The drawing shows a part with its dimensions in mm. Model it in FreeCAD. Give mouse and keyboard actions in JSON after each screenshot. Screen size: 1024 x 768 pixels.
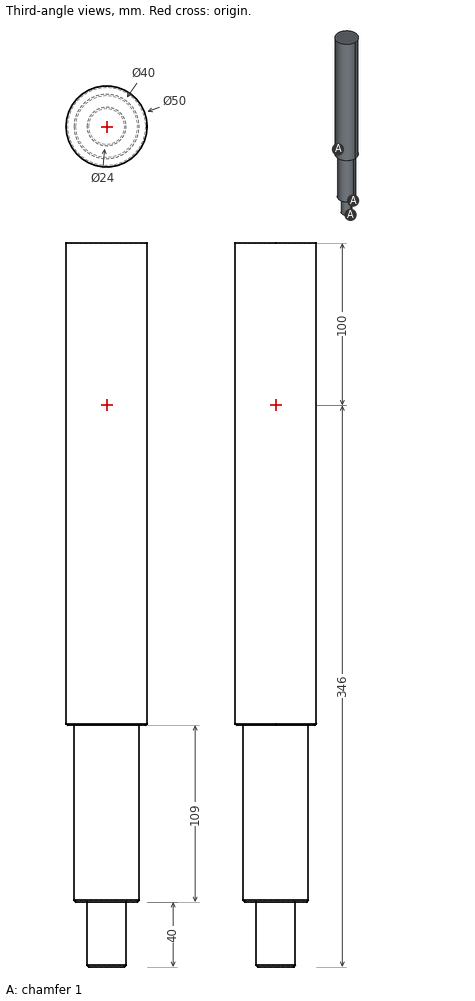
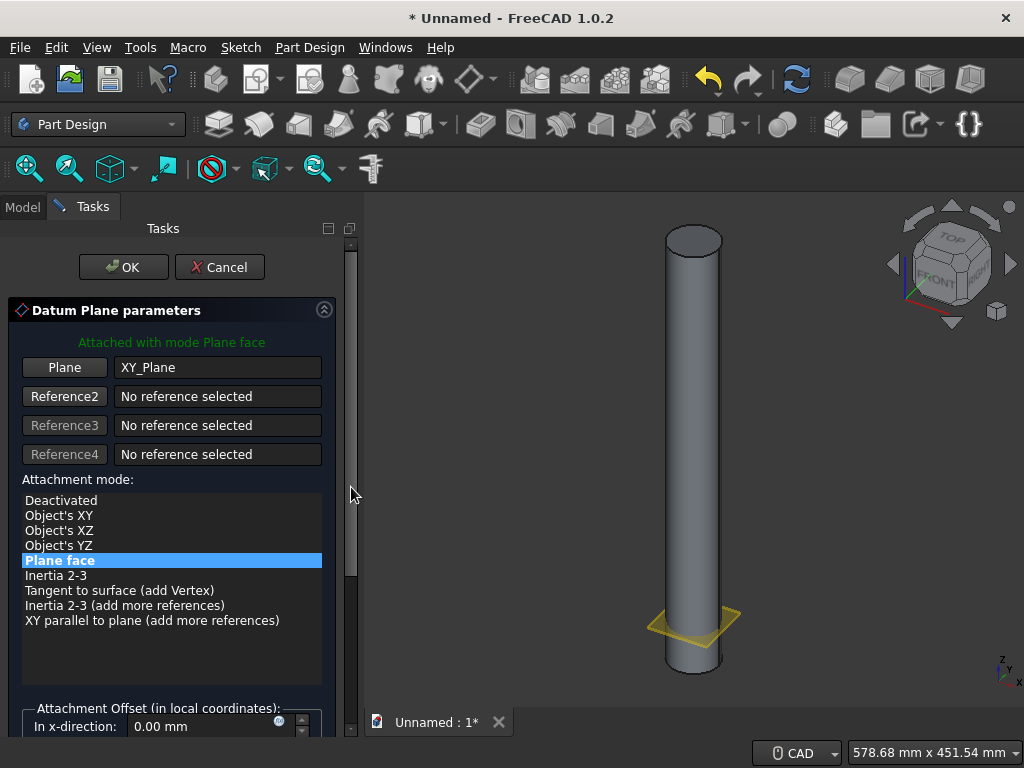
{"action": "left_click", "coordinate": [124, 267]}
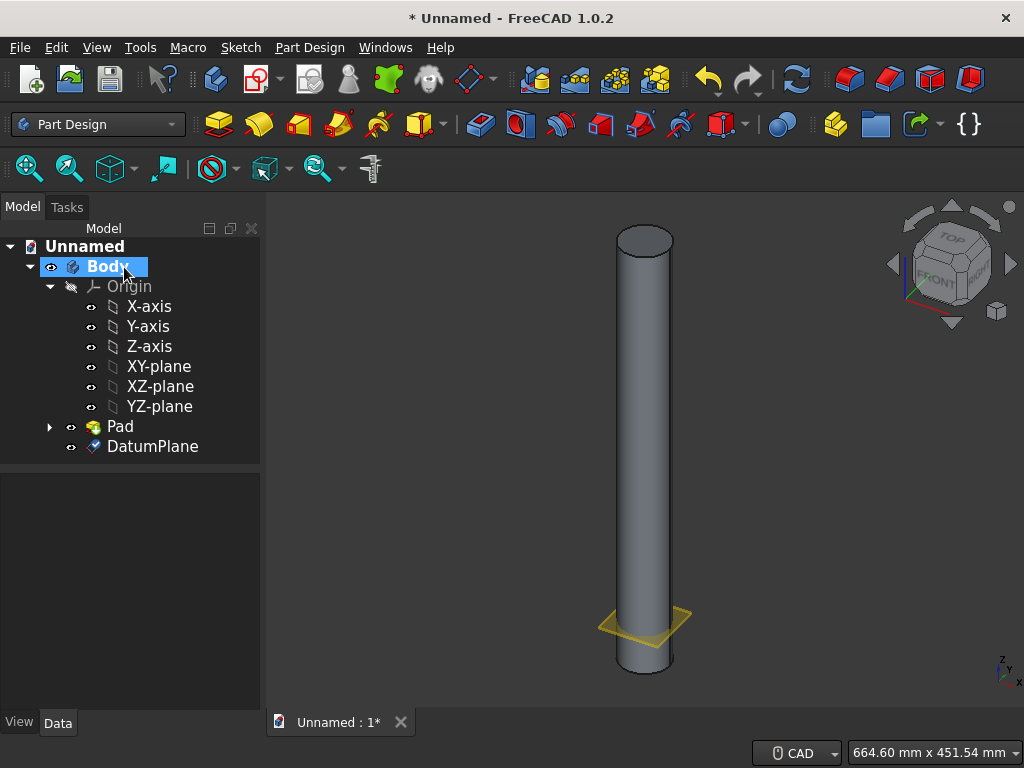
{"action": "left_click", "coordinate": [116, 447]}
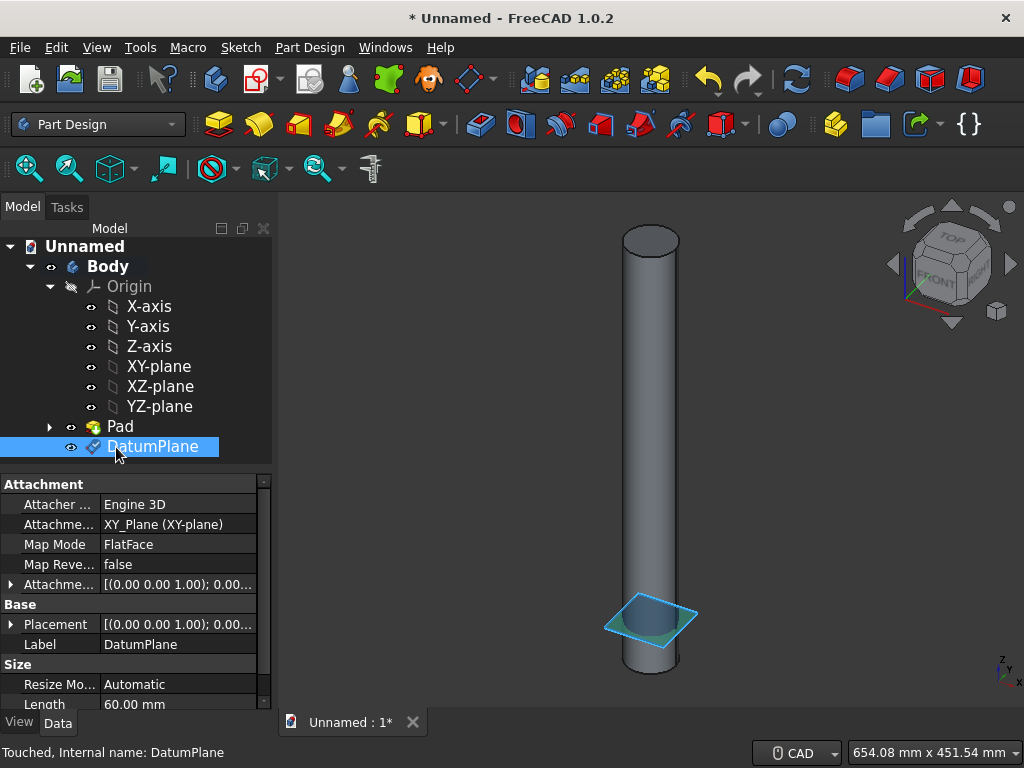
{"action": "left_click", "coordinate": [256, 80]}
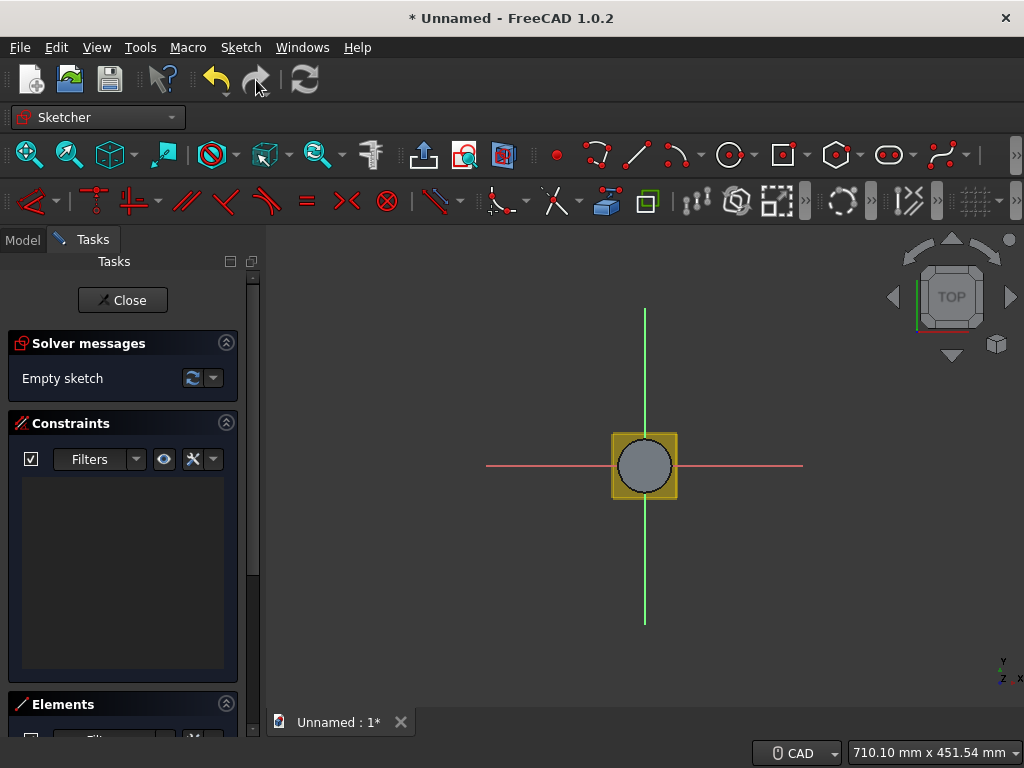
{"action": "left_click", "coordinate": [504, 156]}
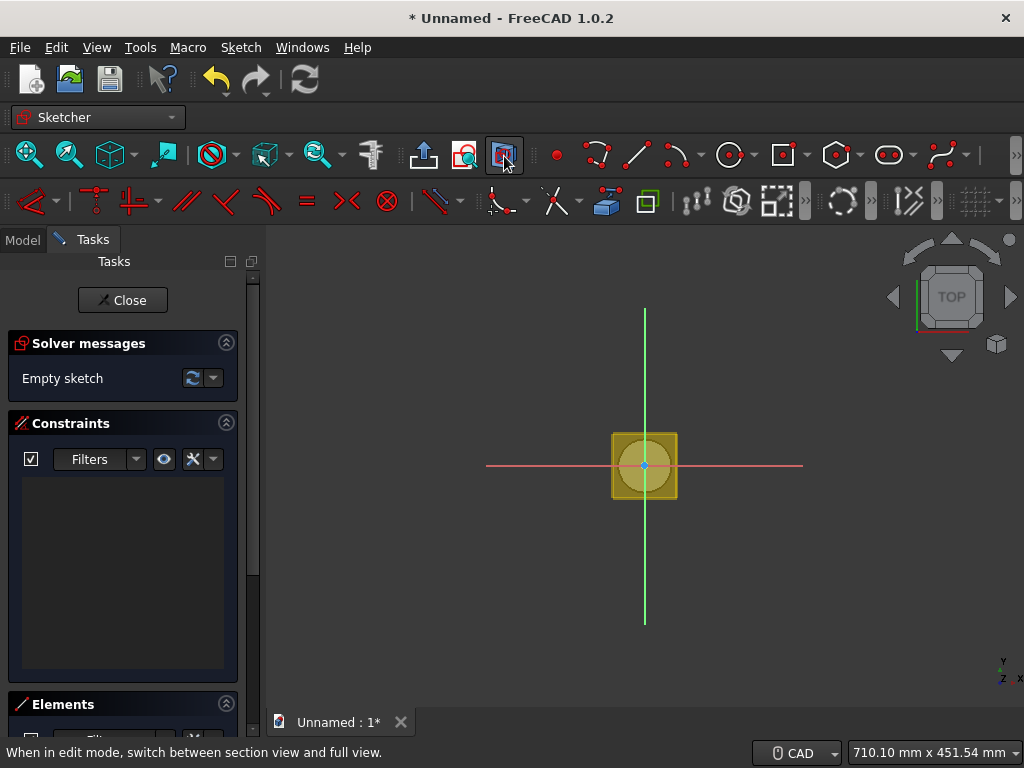
{"action": "scroll", "coordinate": [658, 466], "scroll_direction": "up", "scroll_amount": 9}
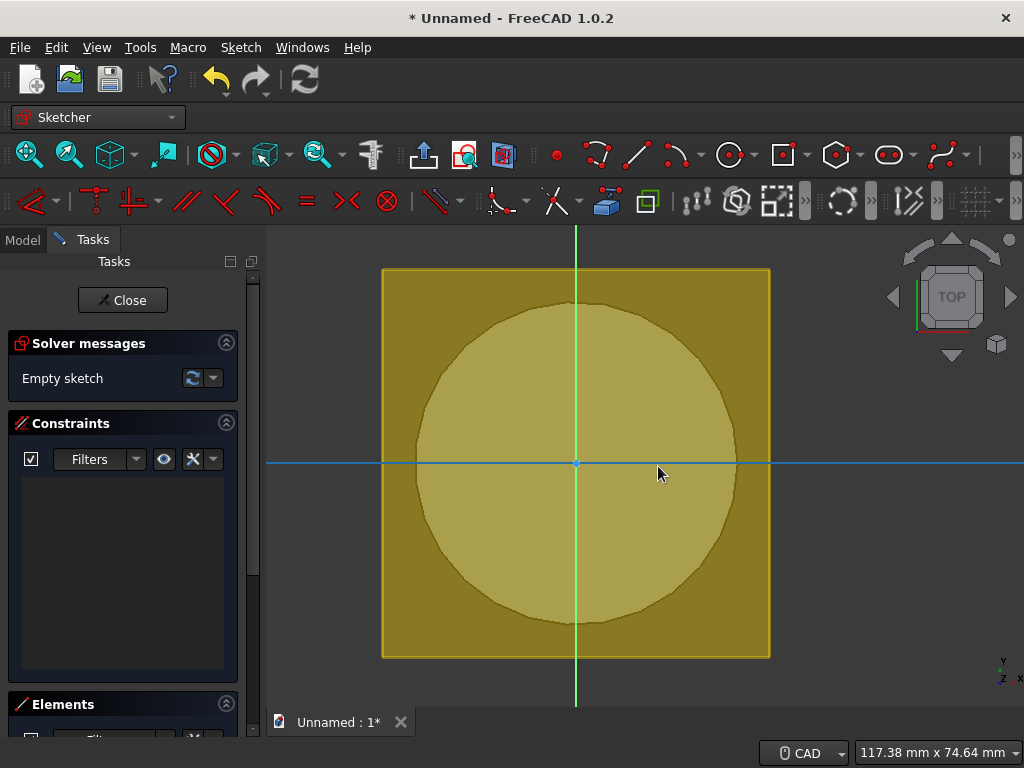
{"action": "left_click", "coordinate": [730, 156]}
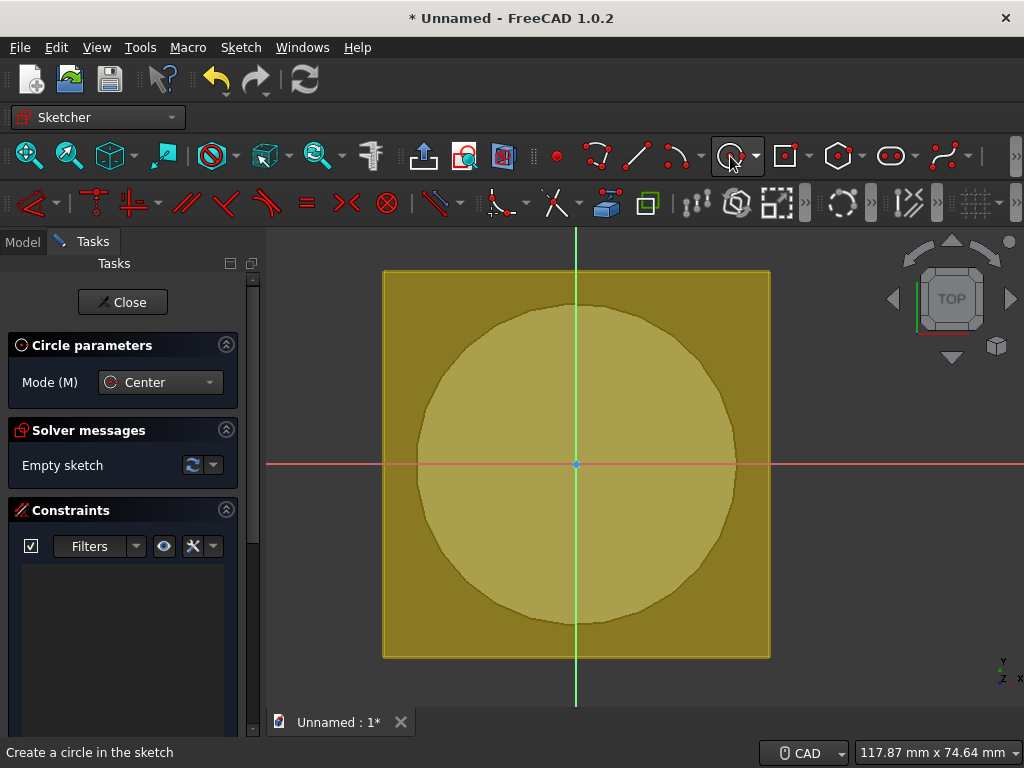
{"action": "left_click", "coordinate": [576, 464]}
{"action": "left_click", "coordinate": [690, 351]}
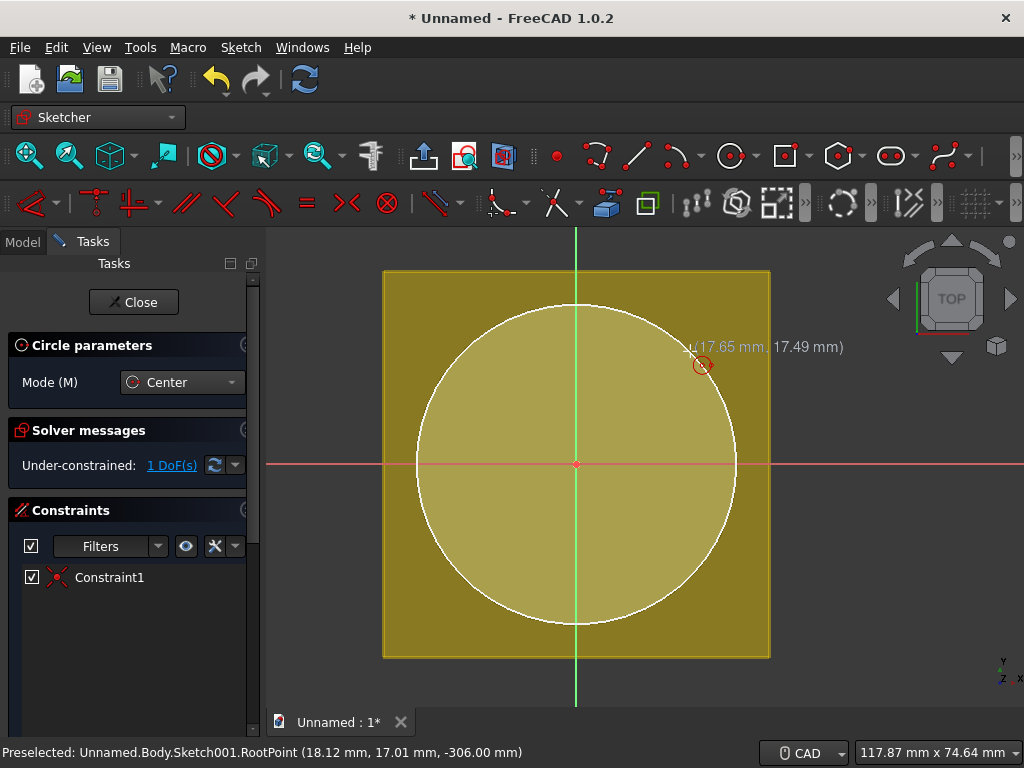
{"action": "left_click", "coordinate": [576, 464]}
{"action": "left_click", "coordinate": [667, 374]}
{"action": "key", "text": "Escape"}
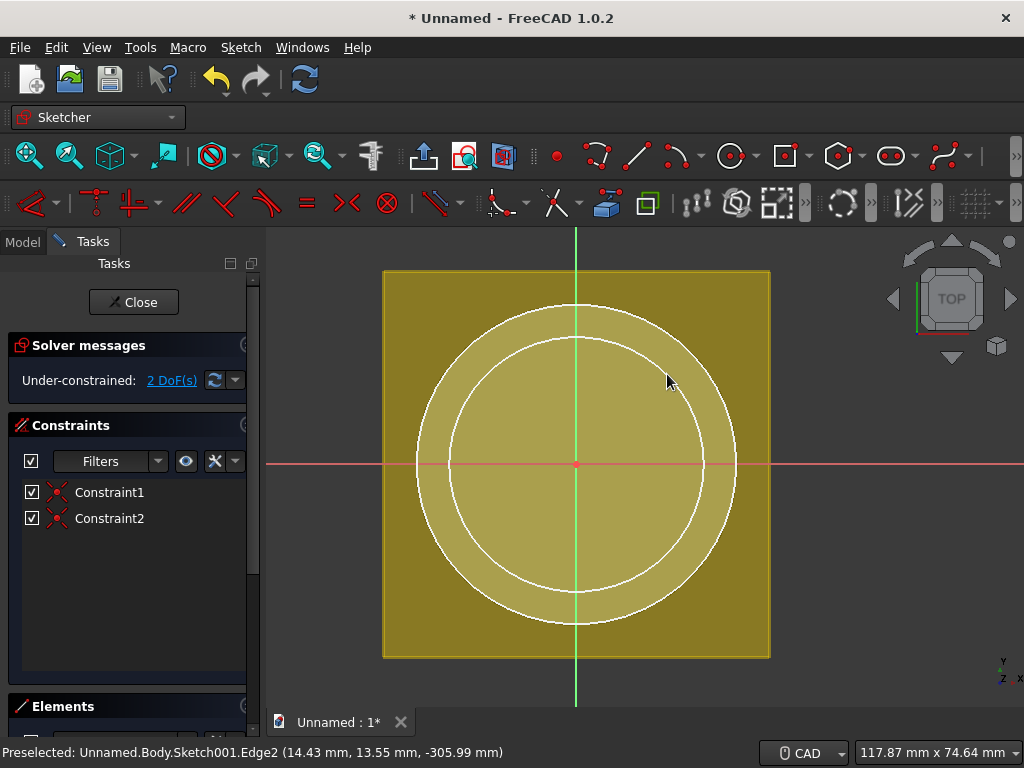
{"action": "key", "text": "d"}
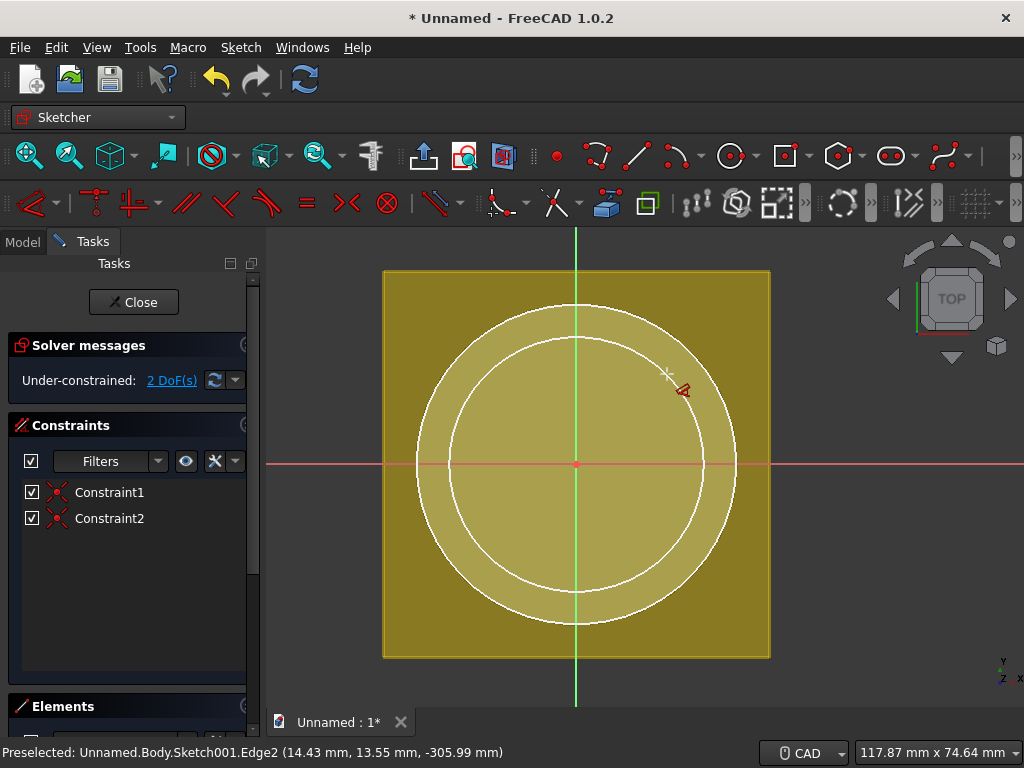
{"action": "left_click", "coordinate": [689, 351]}
{"action": "left_click", "coordinate": [712, 328]}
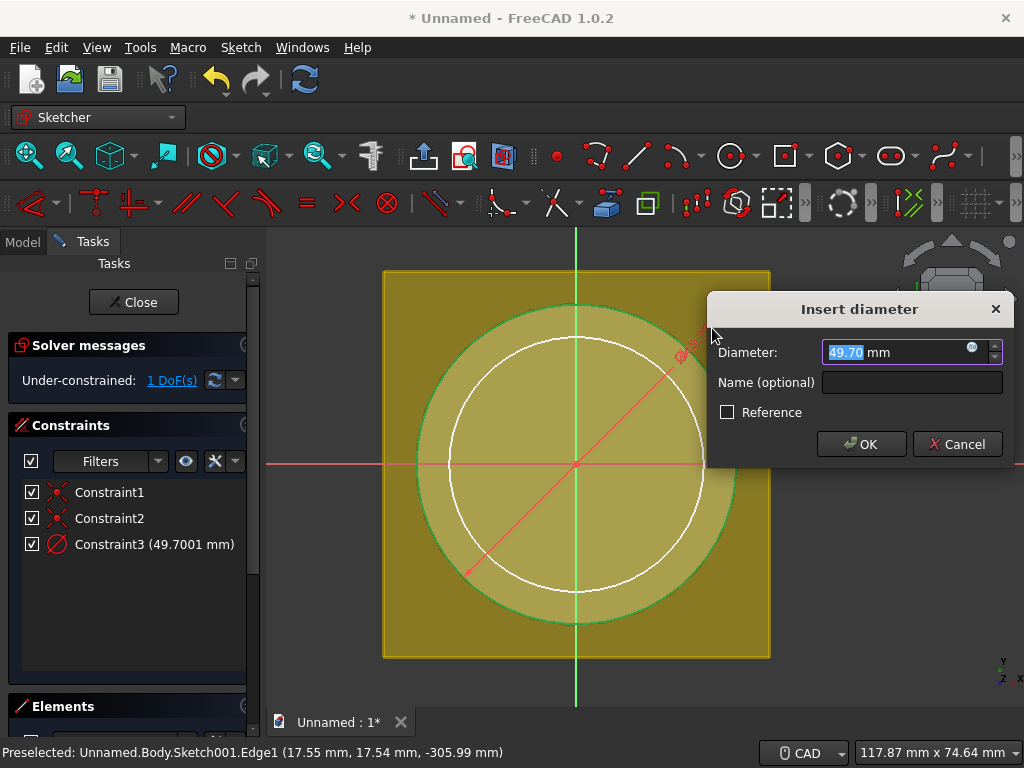
{"action": "type", "text": "50"}
{"action": "key", "text": "Return"}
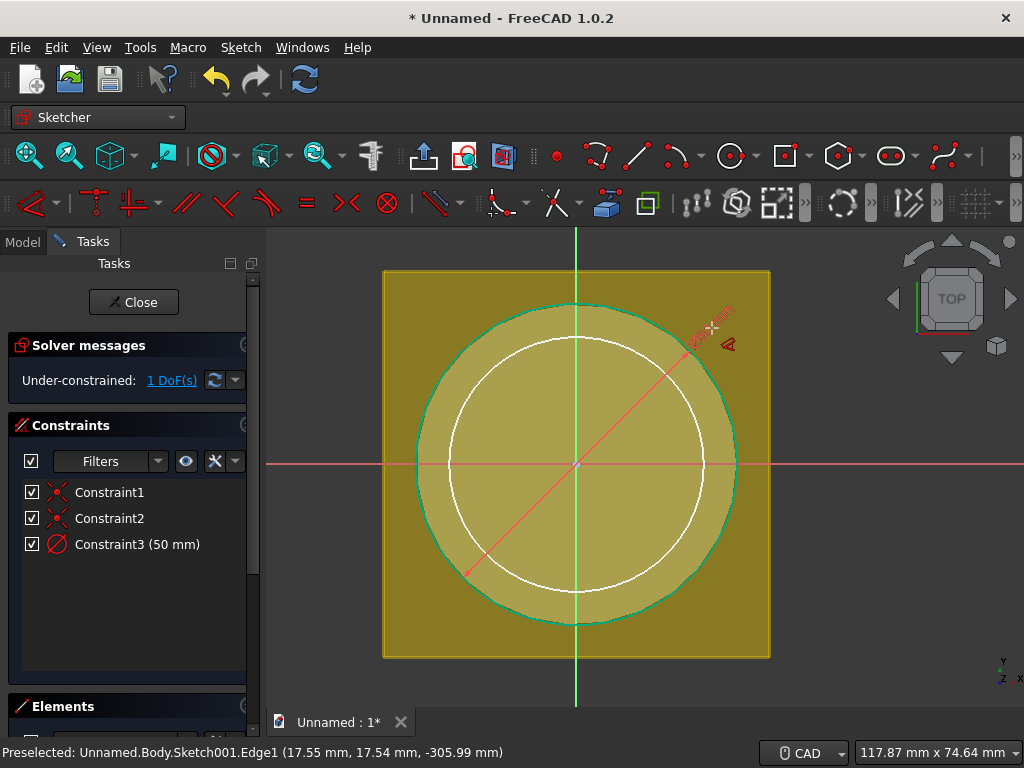
{"action": "left_click", "coordinate": [666, 374]}
{"action": "left_click", "coordinate": [751, 412]}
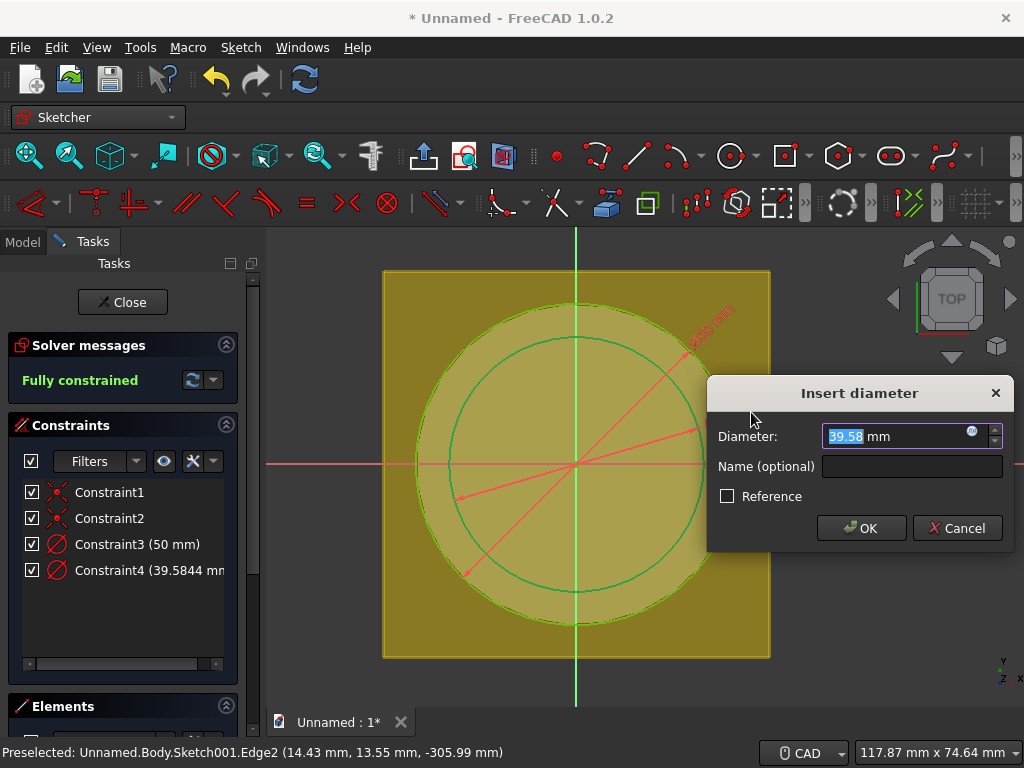
{"action": "type", "text": "40"}
{"action": "key", "text": "Return"}
{"action": "key", "text": "Escape"}